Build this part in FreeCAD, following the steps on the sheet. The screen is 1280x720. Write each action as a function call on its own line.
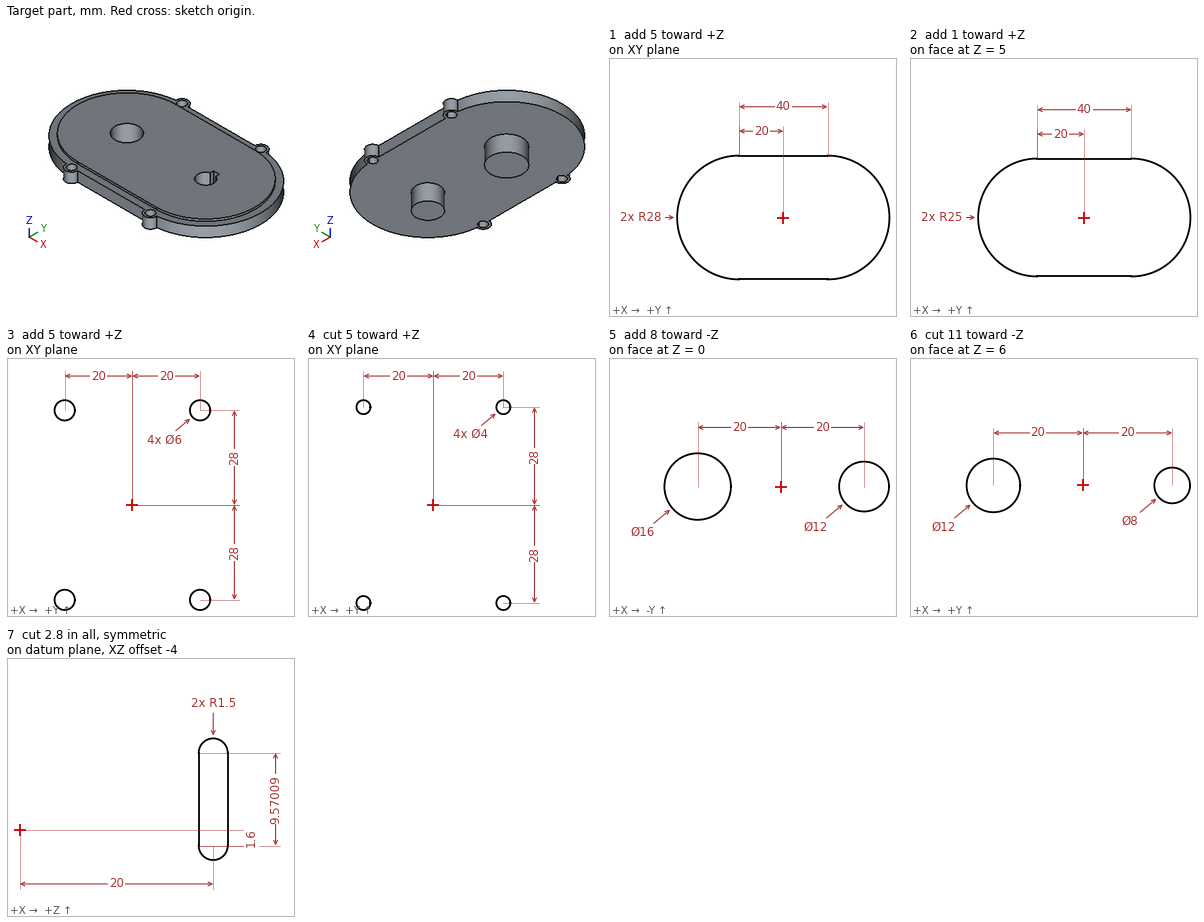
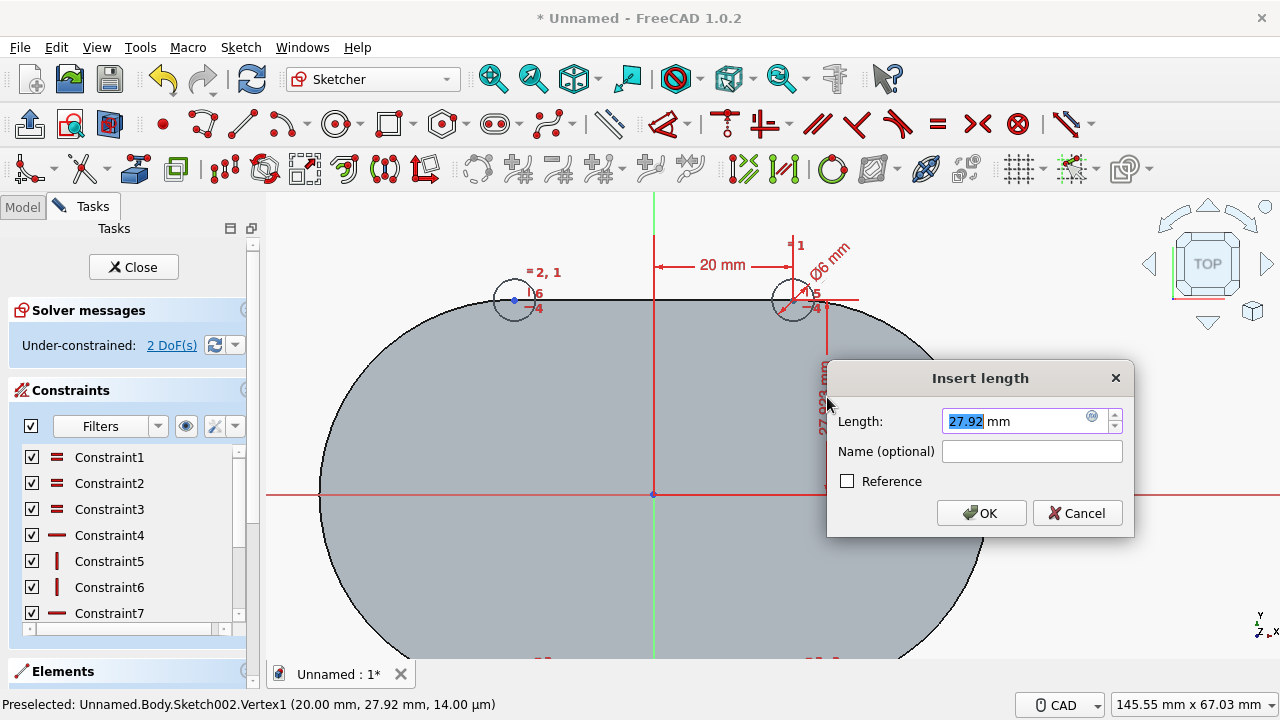
text(28)
key(Return)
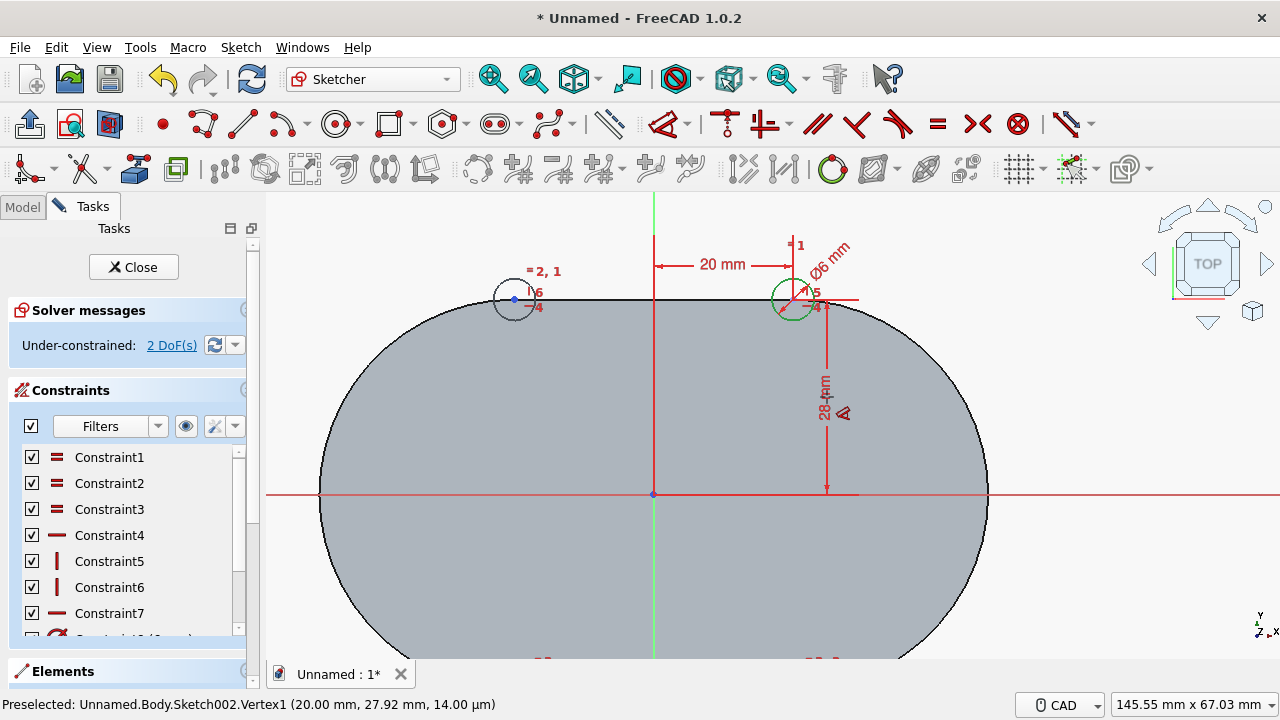
click(515, 300)
click(584, 266)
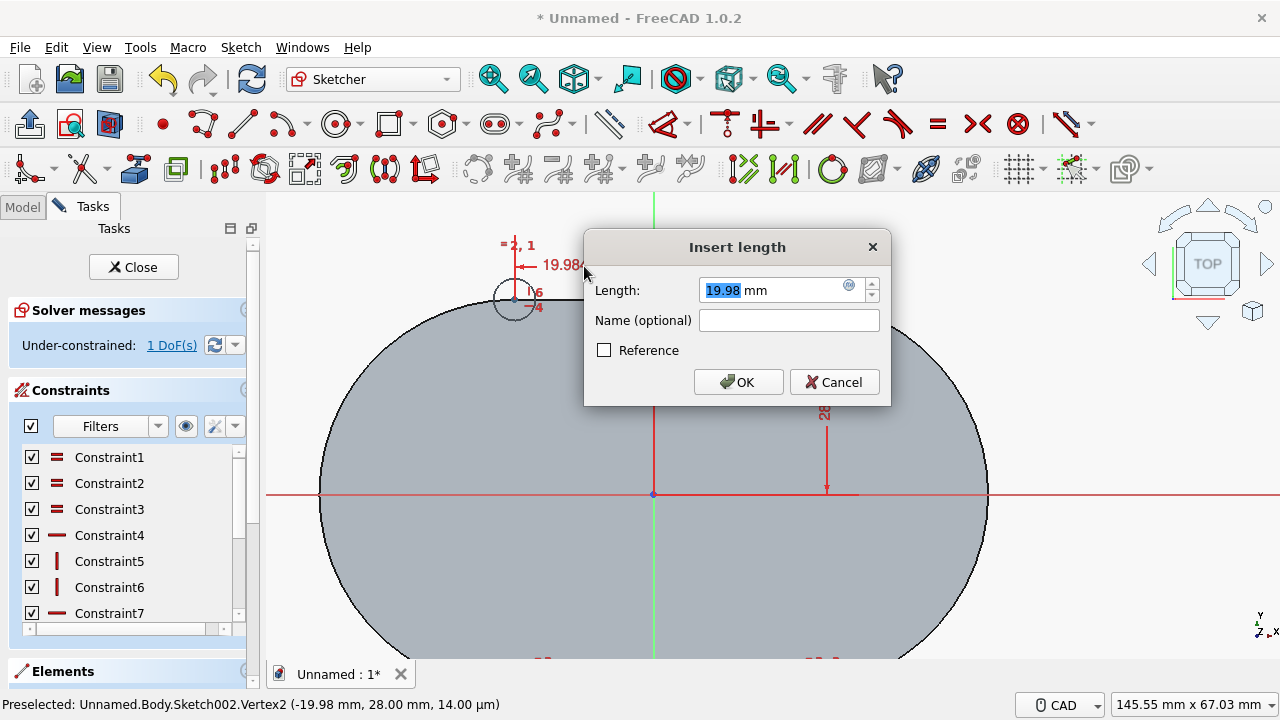
text(20)
key(Return)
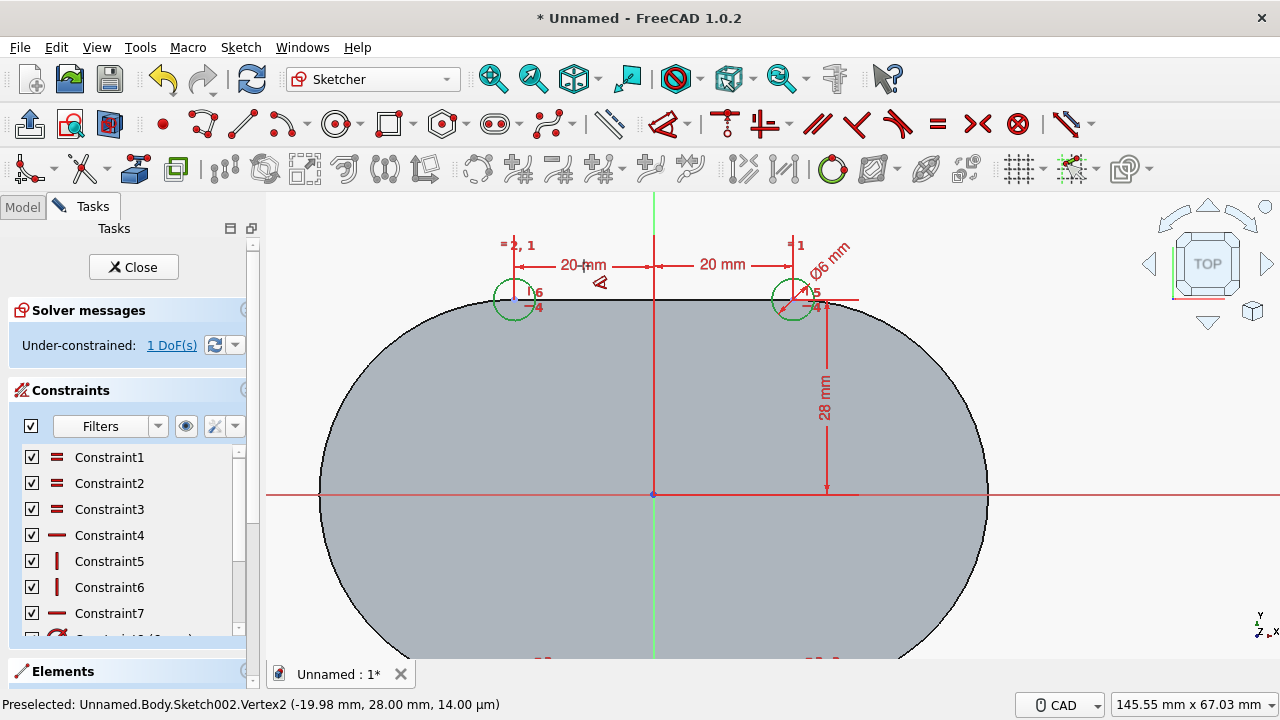
scroll(808, 285, down, 2)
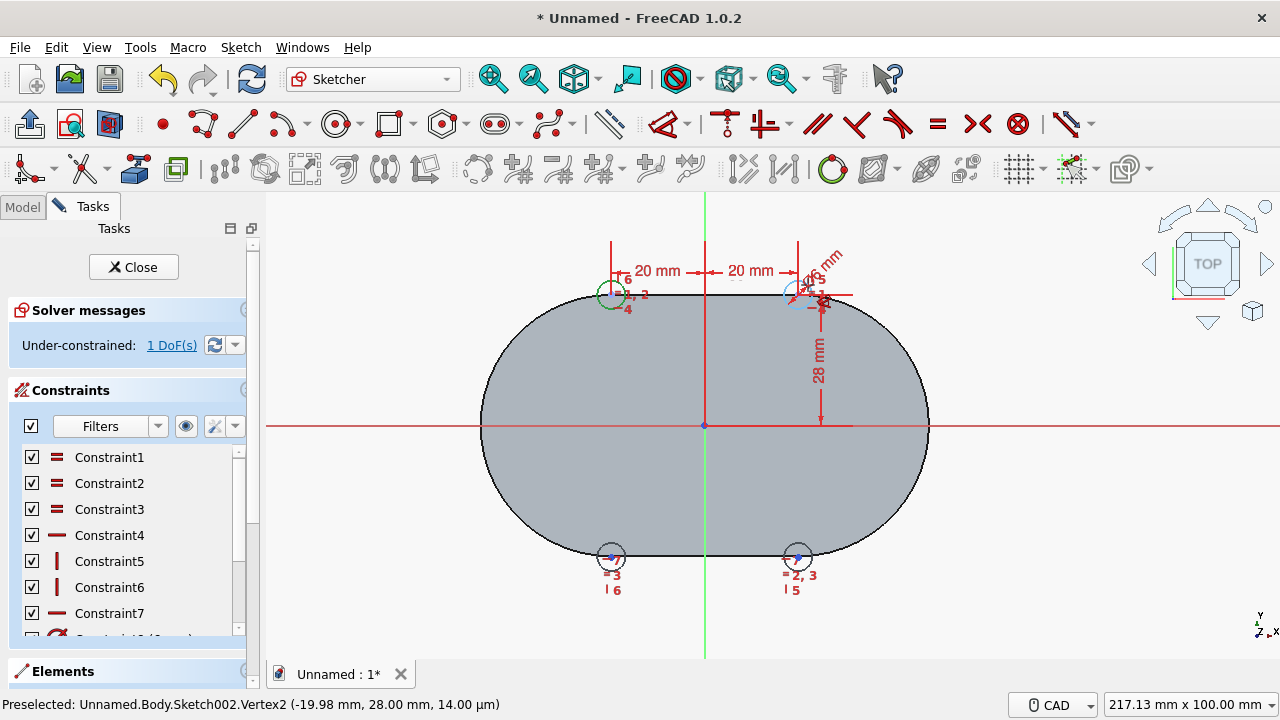
click(798, 557)
click(832, 491)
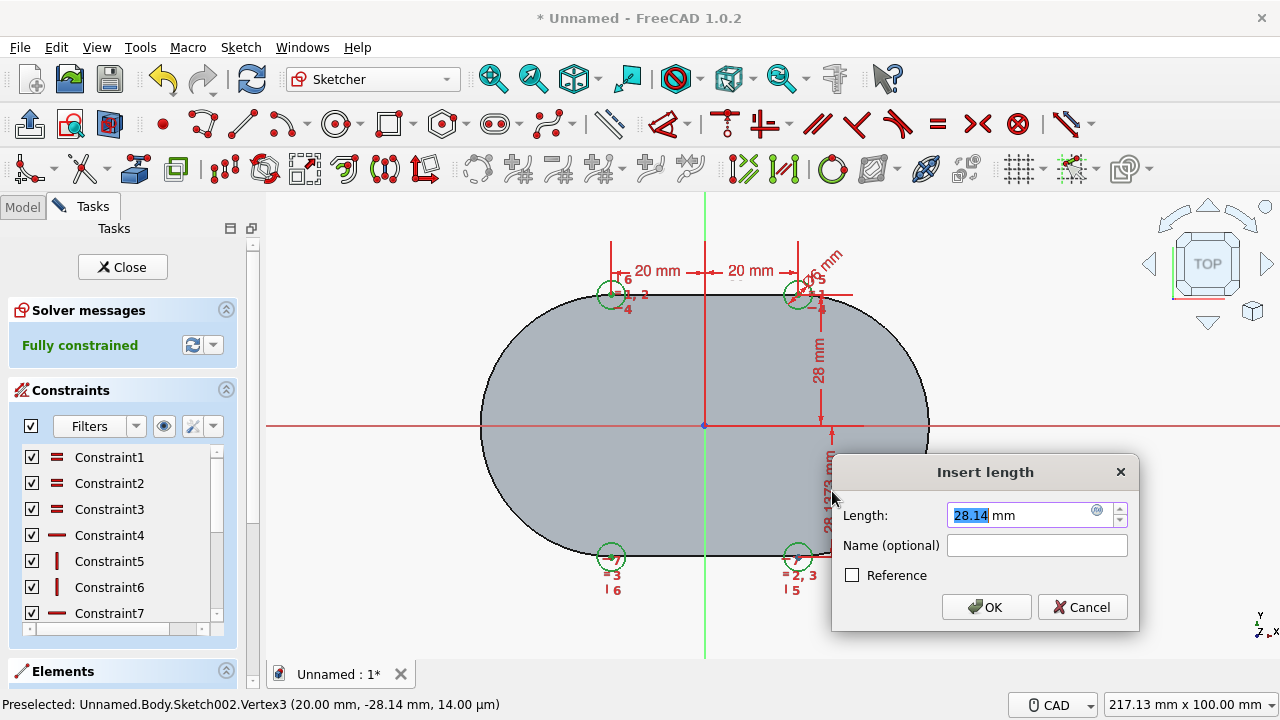
text(28)
key(Return)
key(Escape)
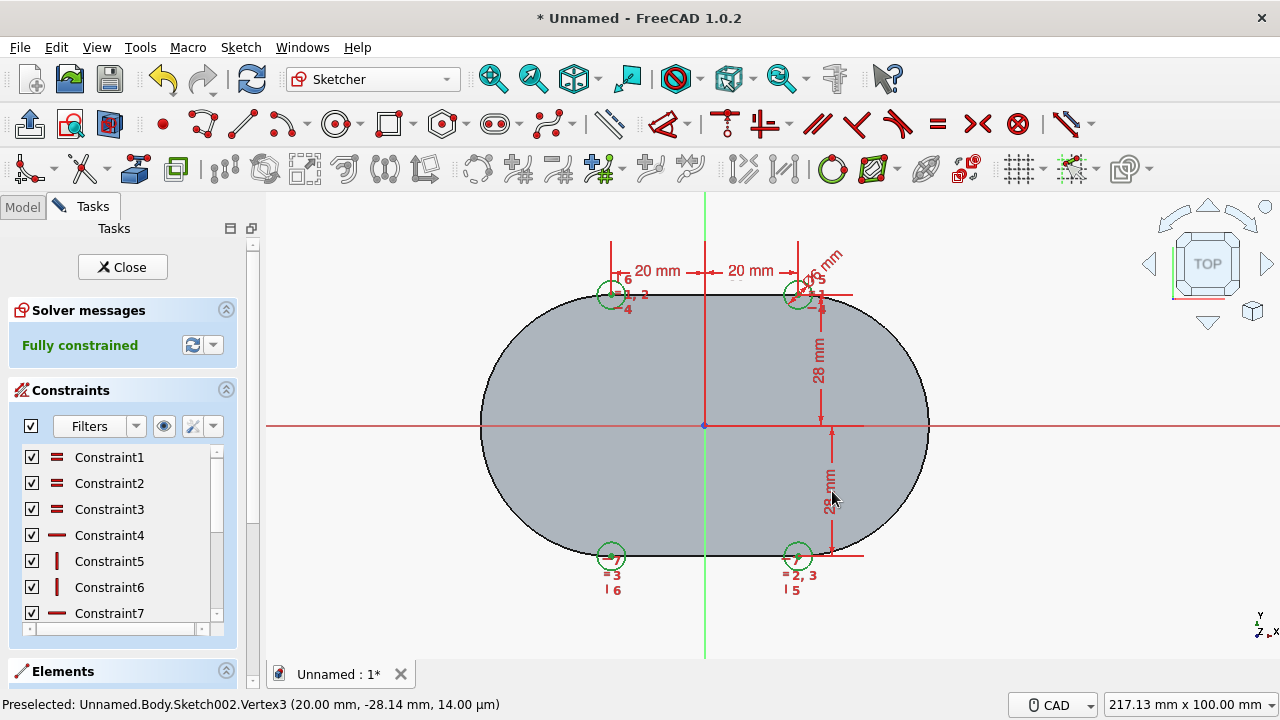
click(123, 267)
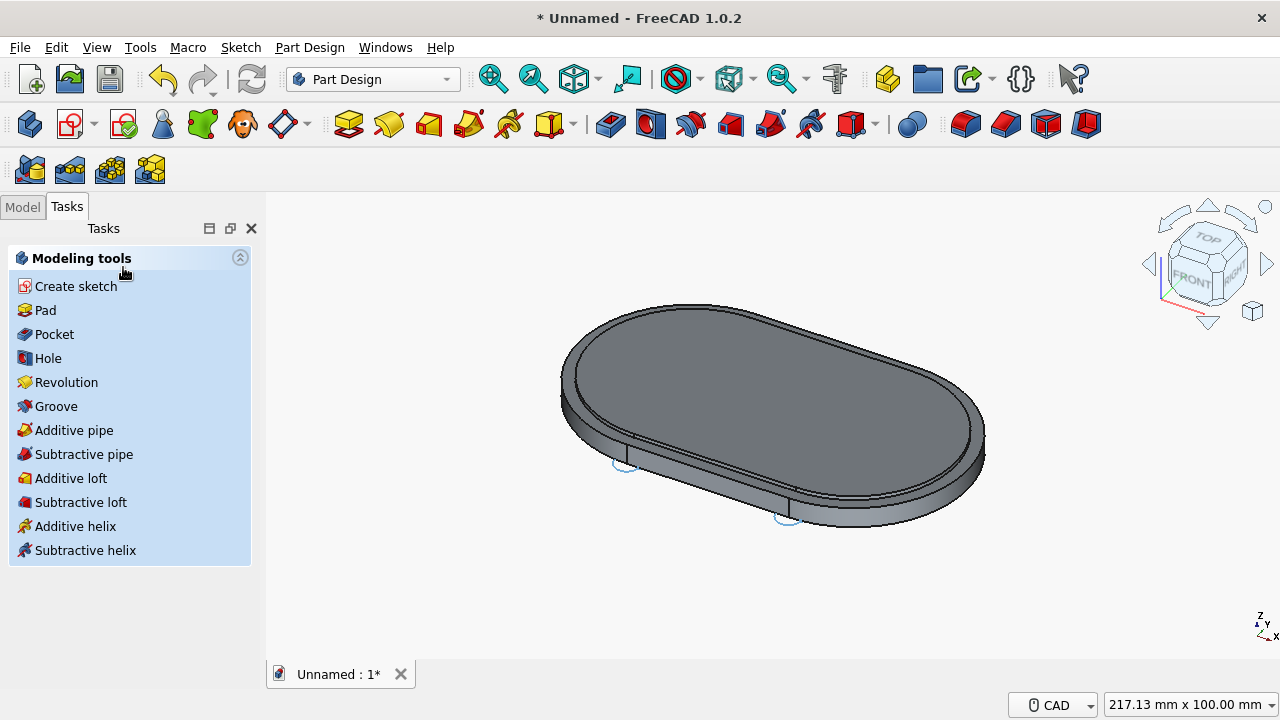
click(350, 124)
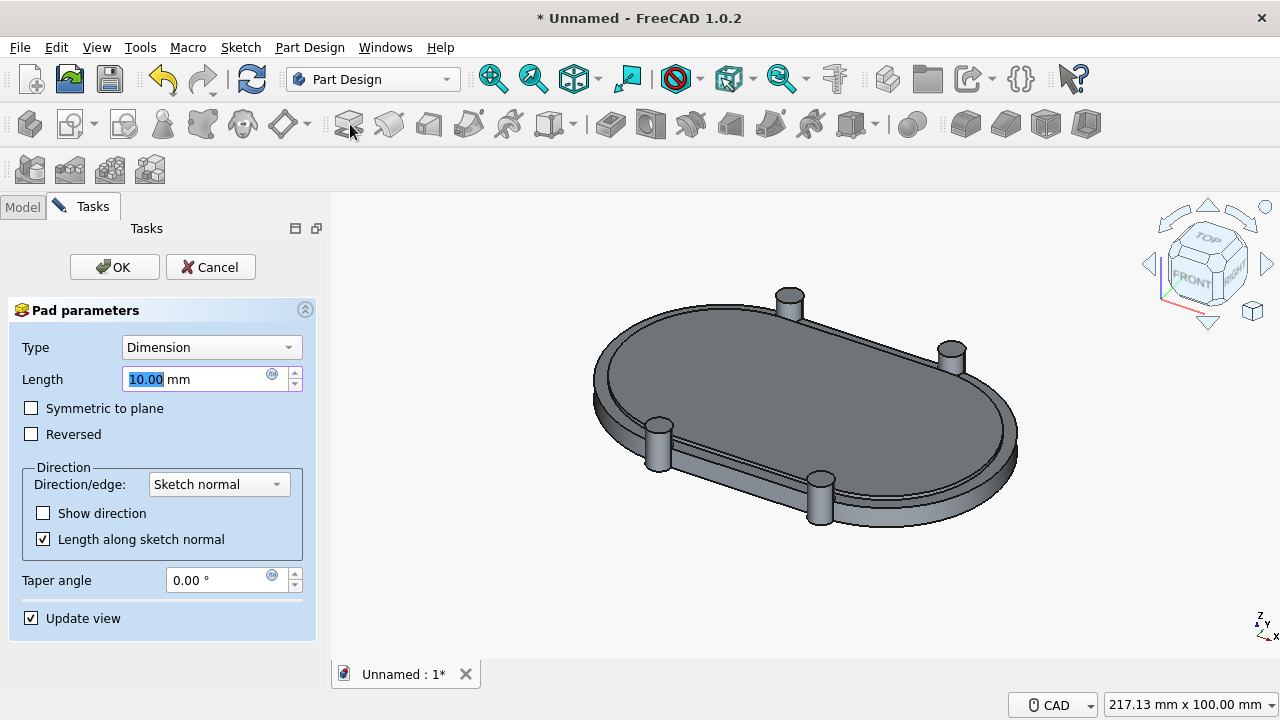
text(5)
key(Tab)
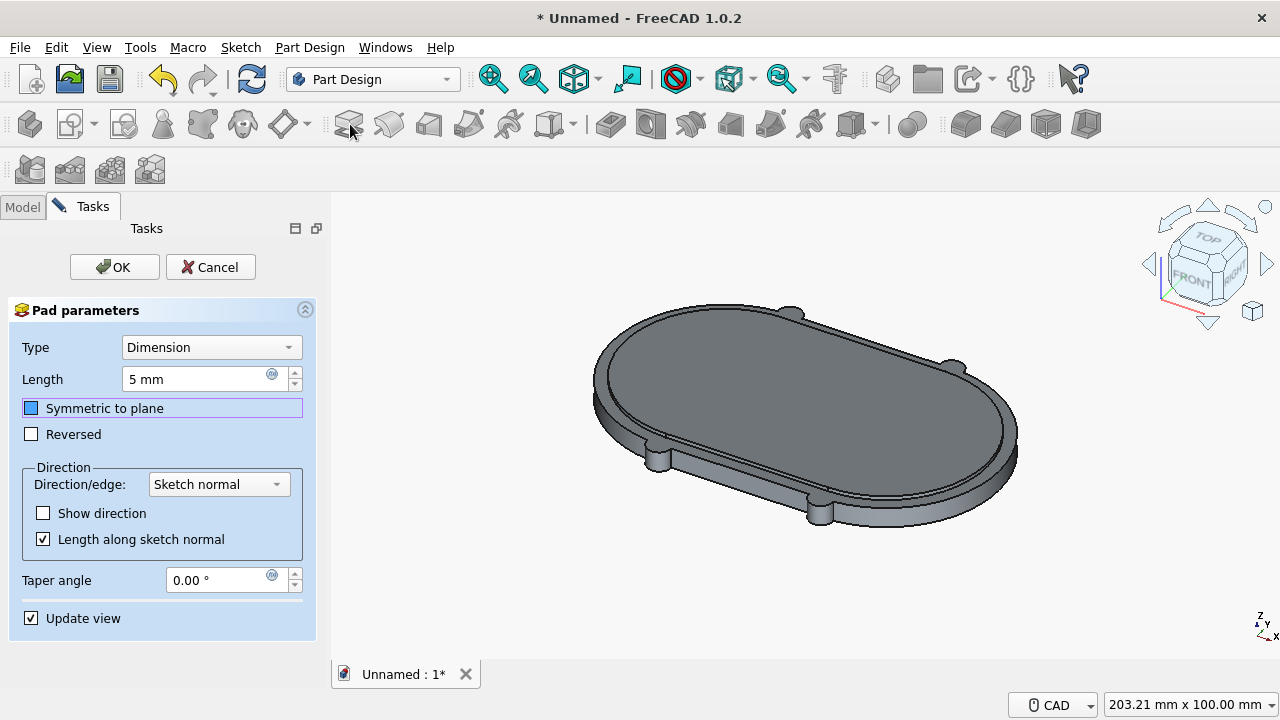
click(115, 267)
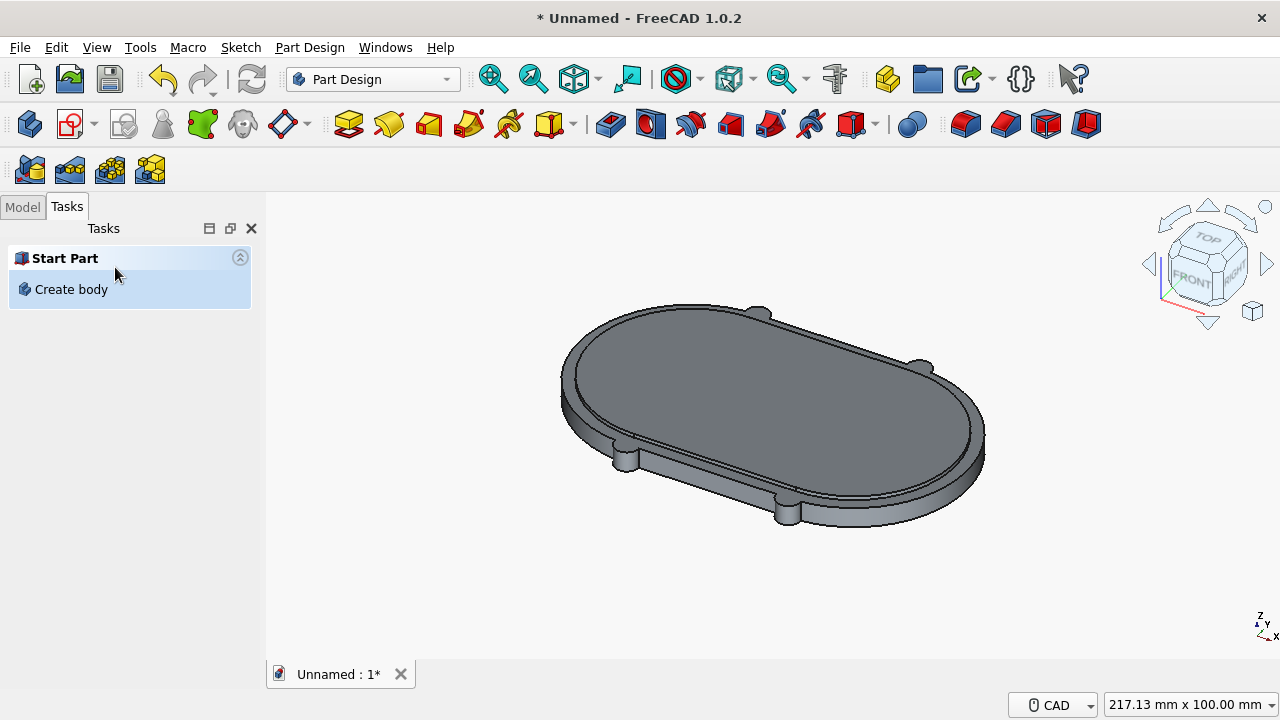
click(70, 124)